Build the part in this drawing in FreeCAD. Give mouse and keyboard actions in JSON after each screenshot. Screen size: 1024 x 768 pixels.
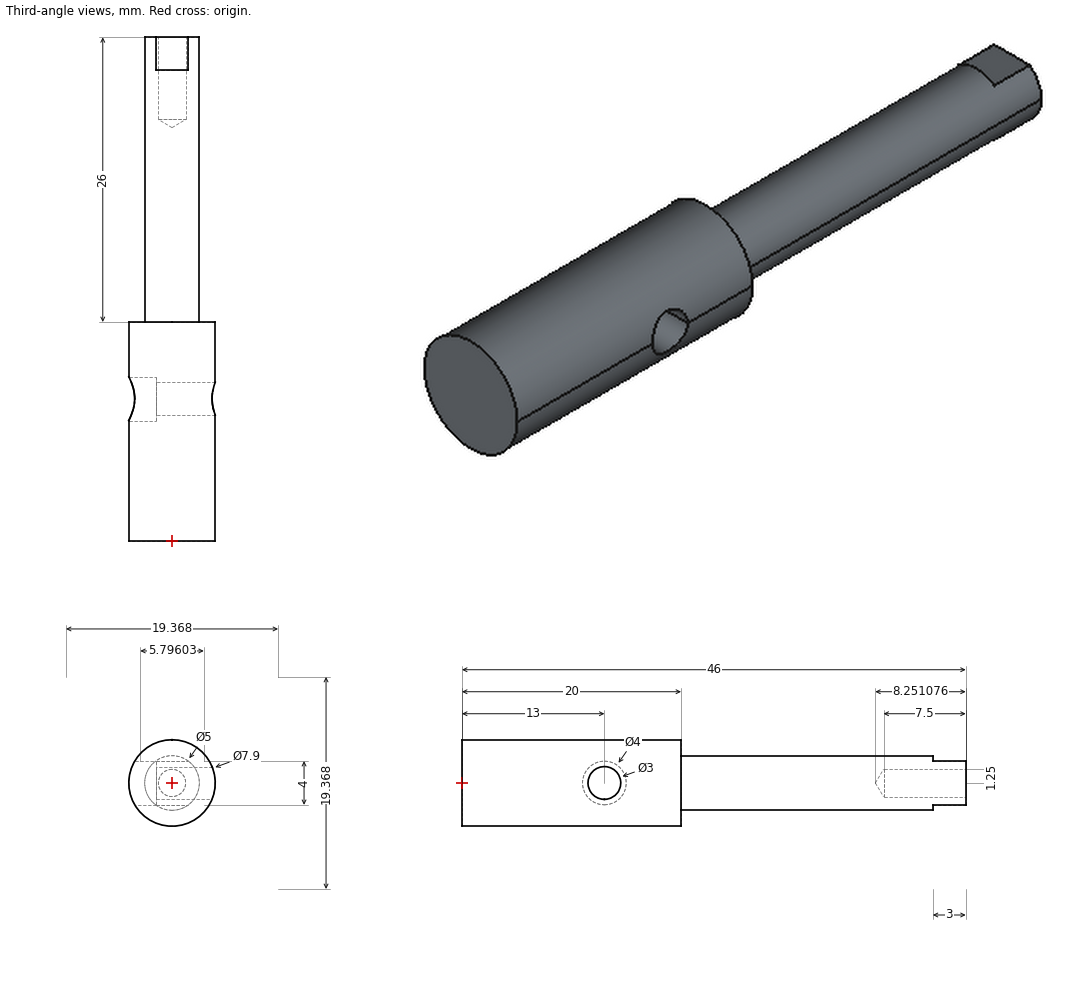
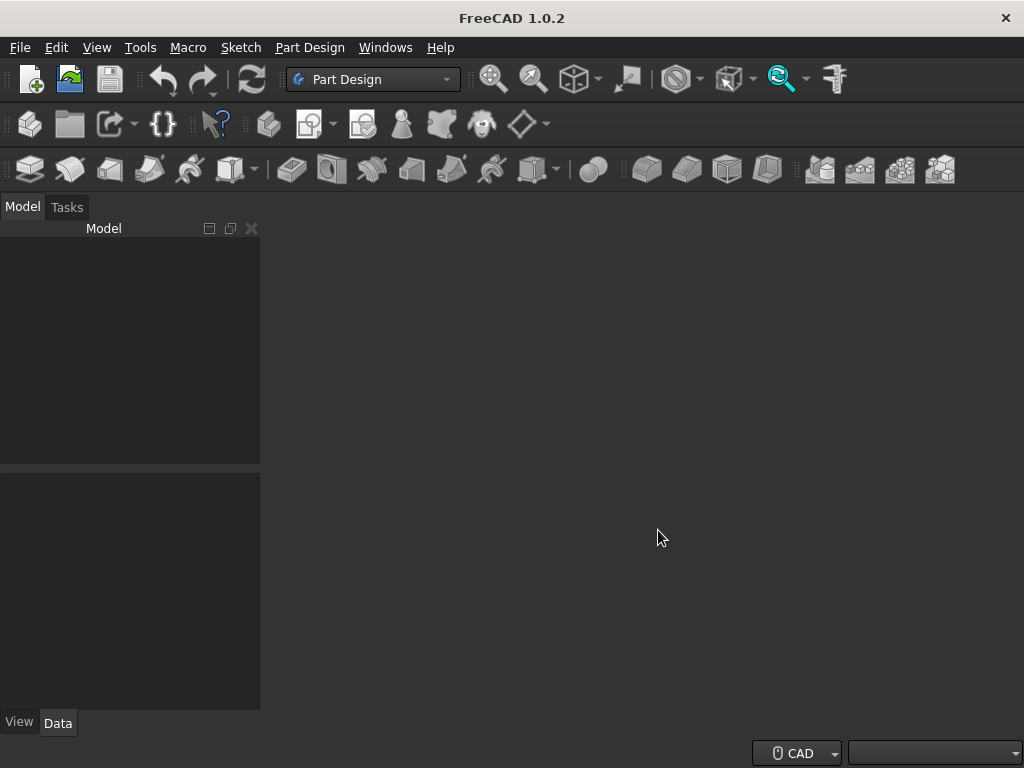
{"action": "left_click", "coordinate": [30, 80]}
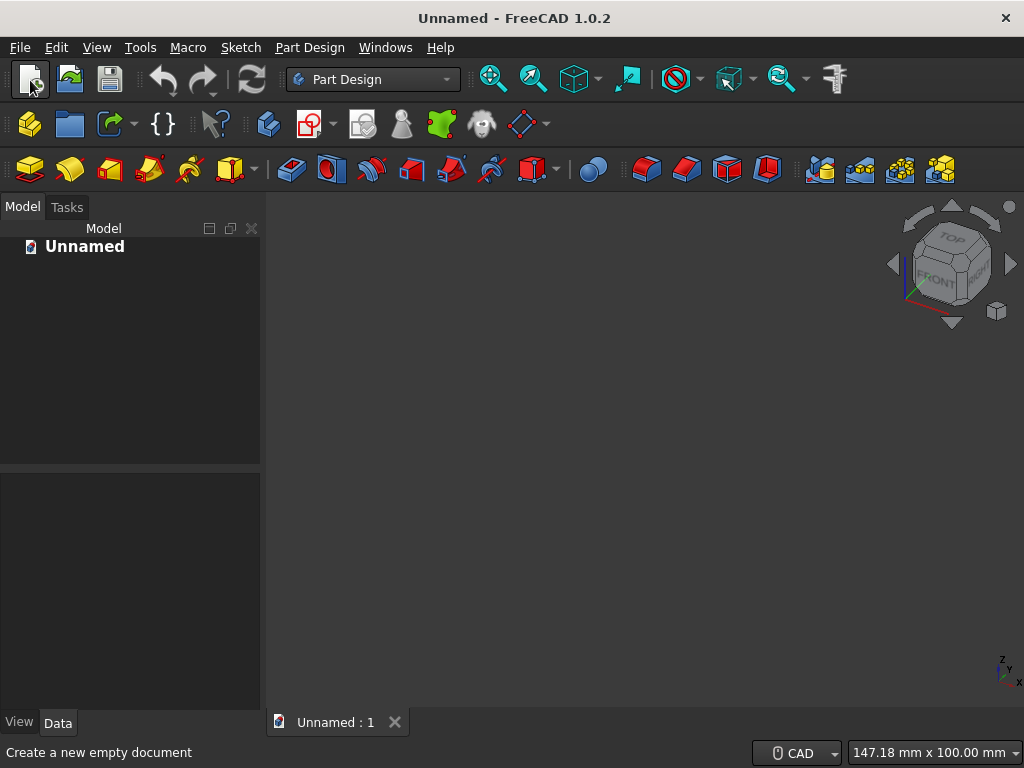
{"action": "left_click", "coordinate": [310, 124]}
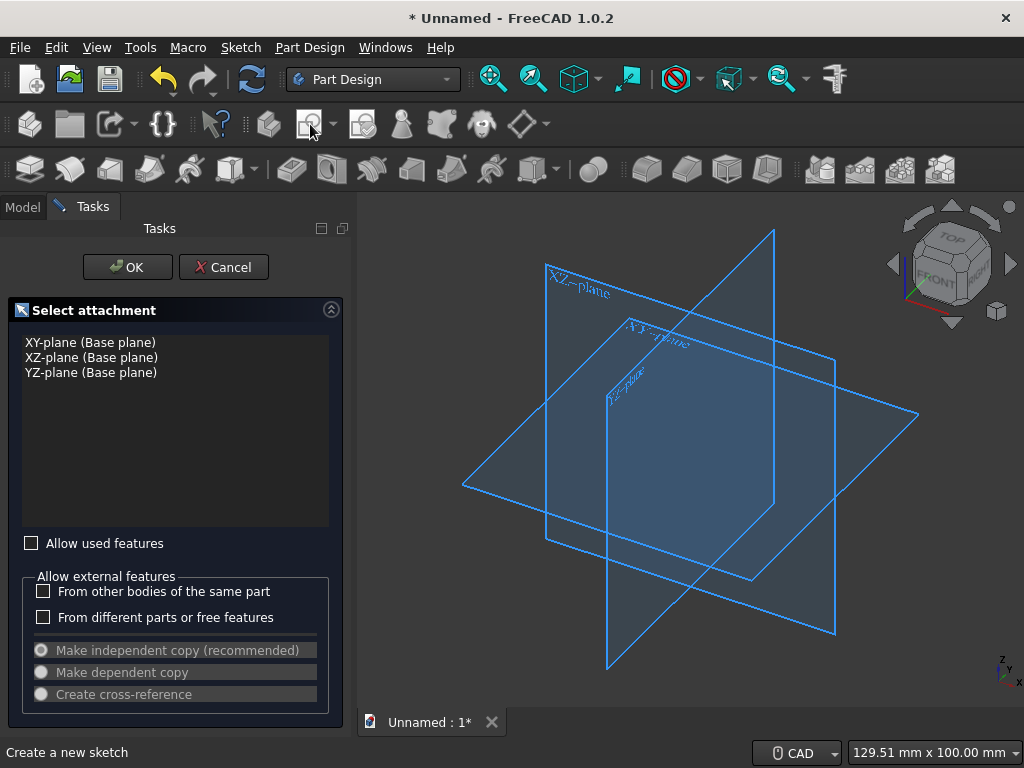
{"action": "left_click", "coordinate": [82, 358]}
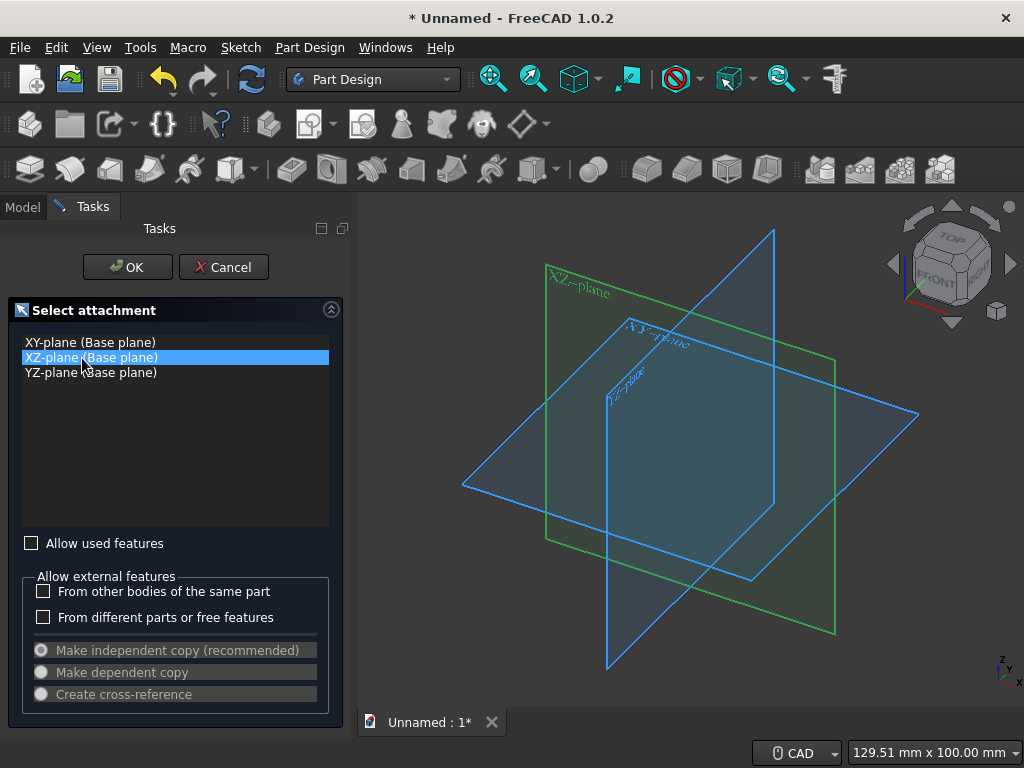
{"action": "left_click", "coordinate": [128, 267]}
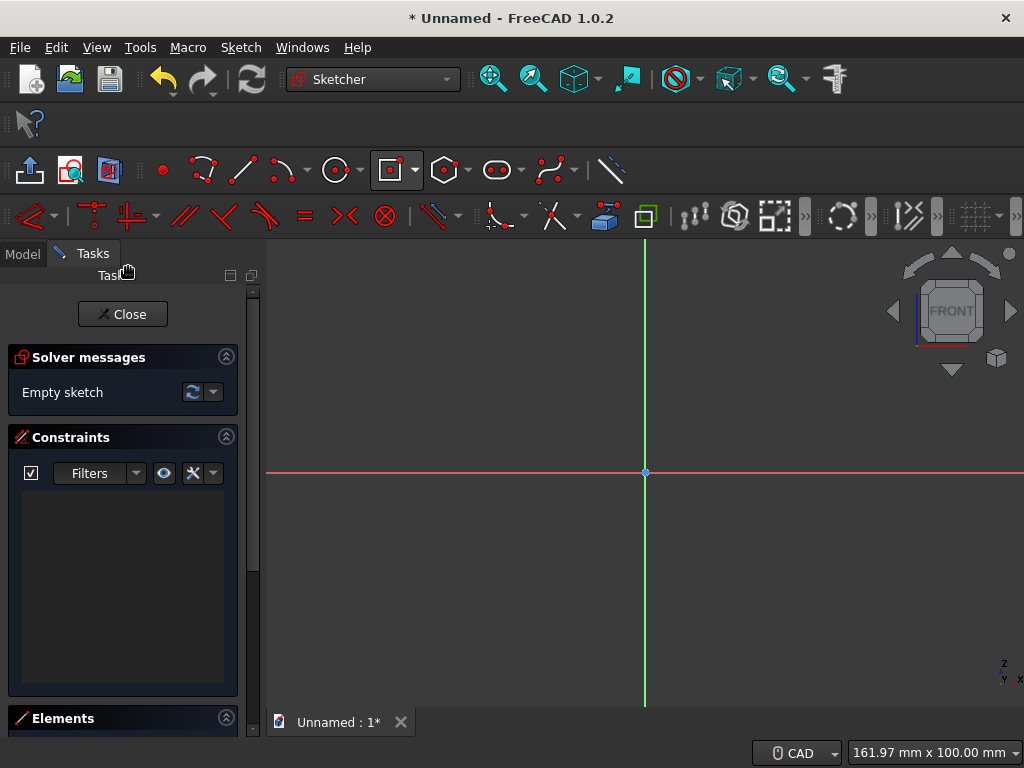
{"action": "scroll", "coordinate": [656, 473], "scroll_direction": "up", "scroll_amount": 10}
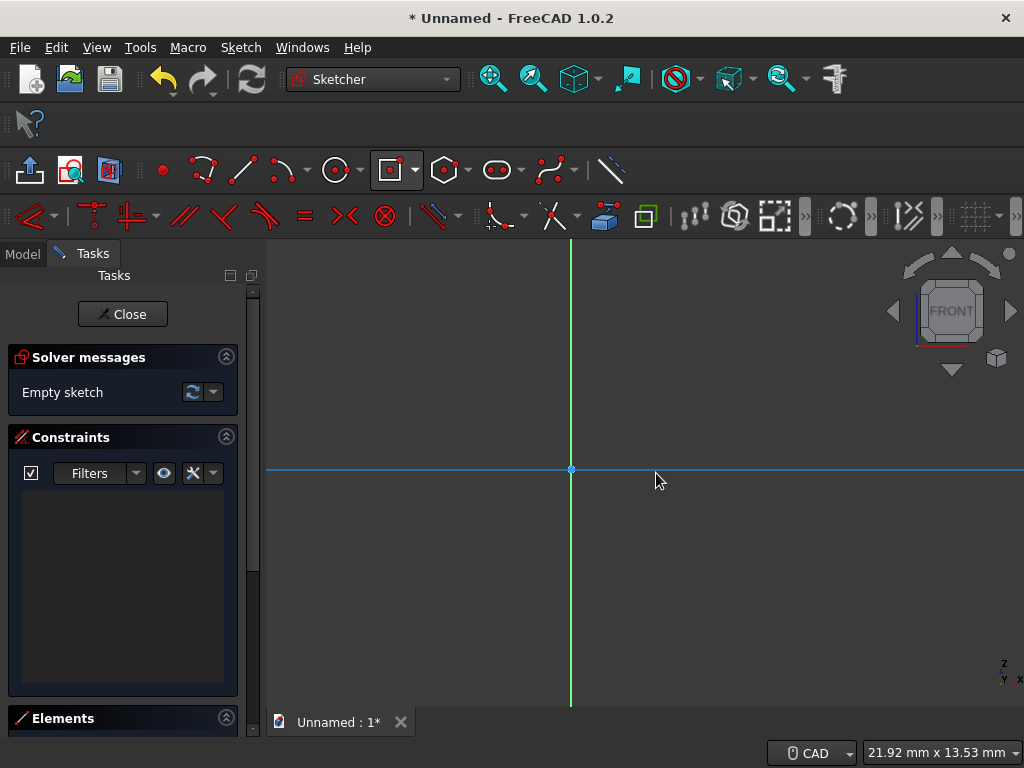
{"action": "left_click", "coordinate": [336, 170]}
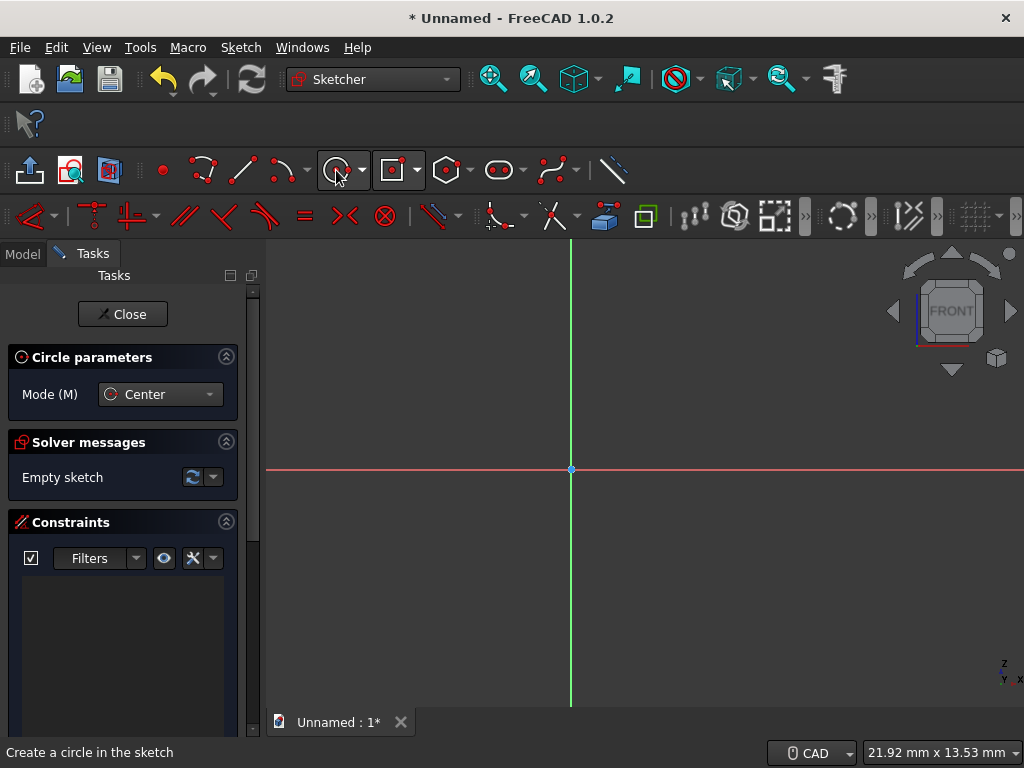
{"action": "left_click", "coordinate": [571, 470]}
{"action": "mouse_move", "coordinate": [668, 373]}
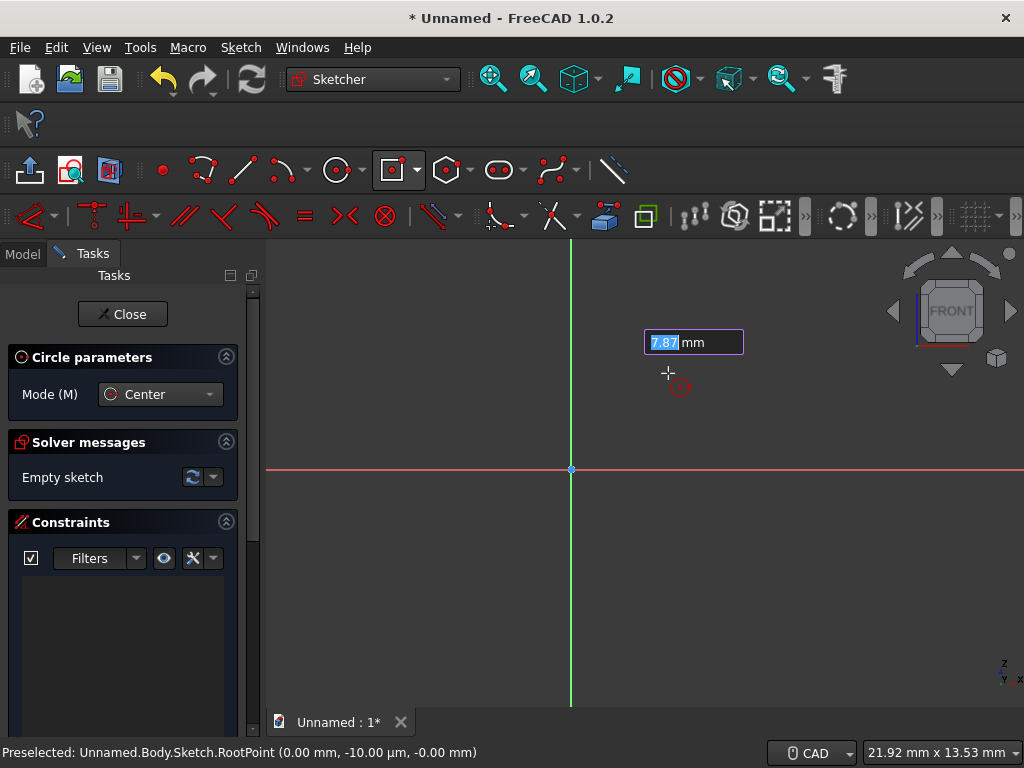
{"action": "type", "text": "7.9"}
{"action": "key", "text": "Return"}
{"action": "key", "text": "Escape"}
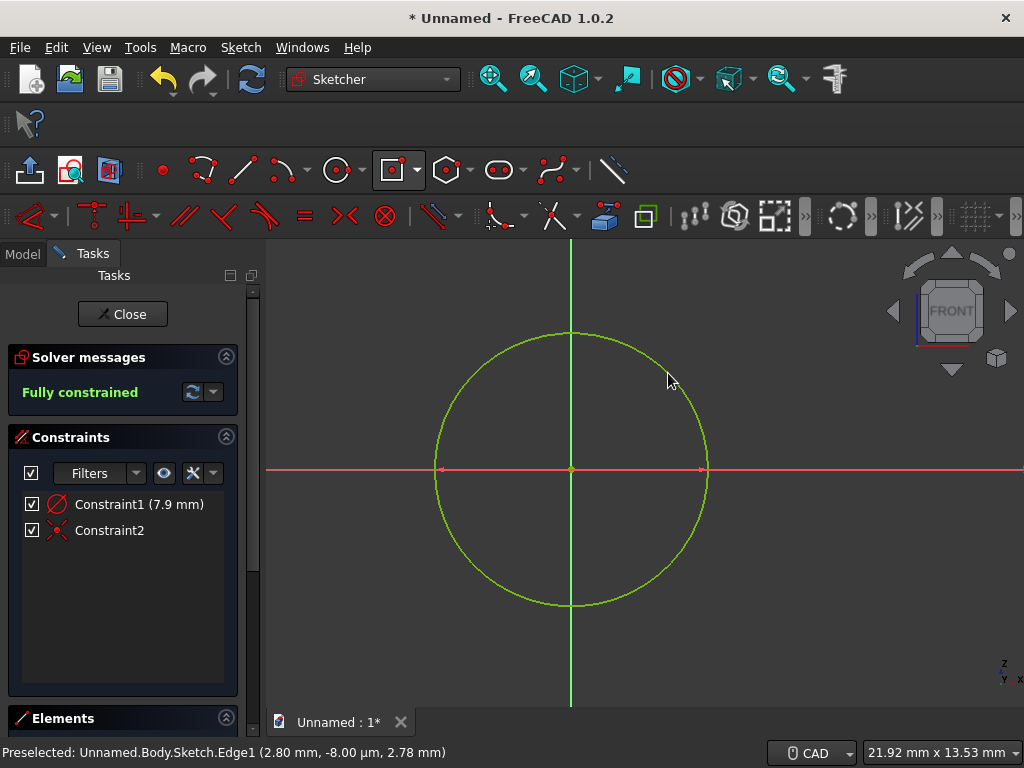
{"action": "left_click", "coordinate": [123, 314]}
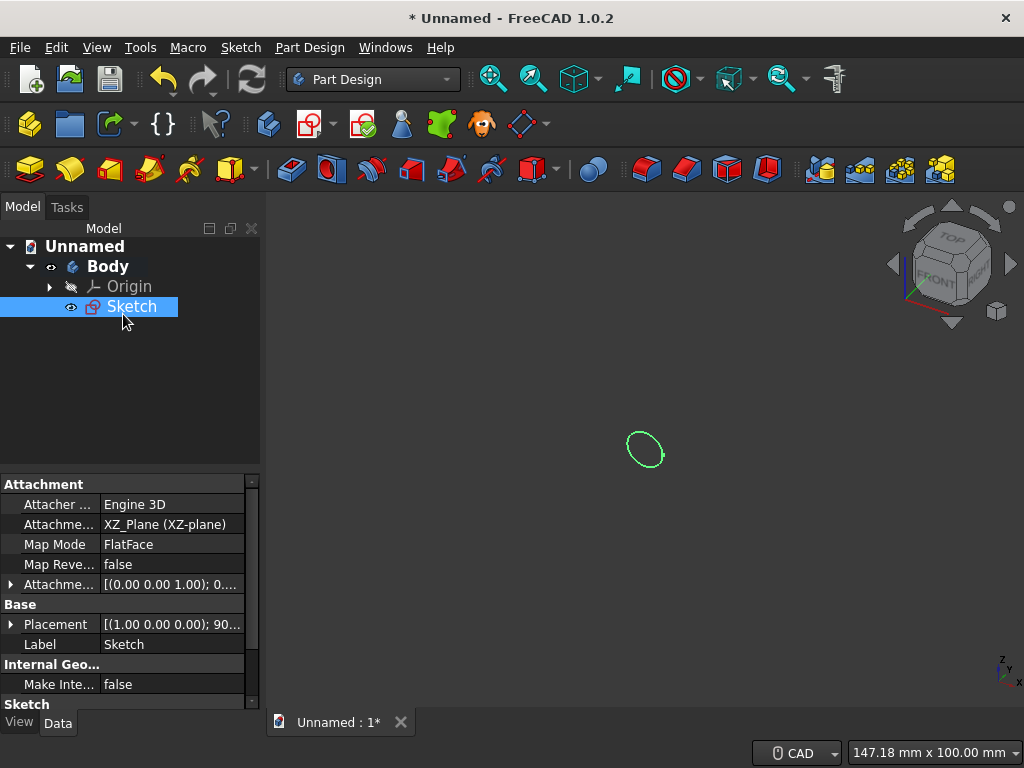
{"action": "left_click", "coordinate": [30, 170]}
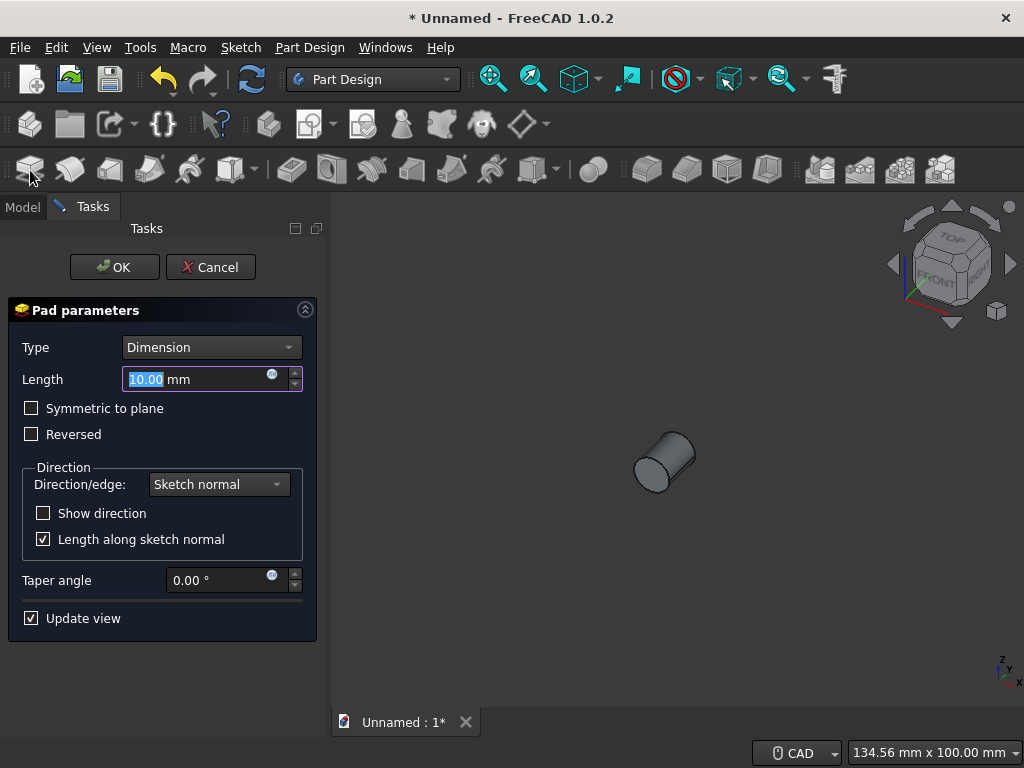
{"action": "type", "text": "20"}
{"action": "key", "text": "Tab"}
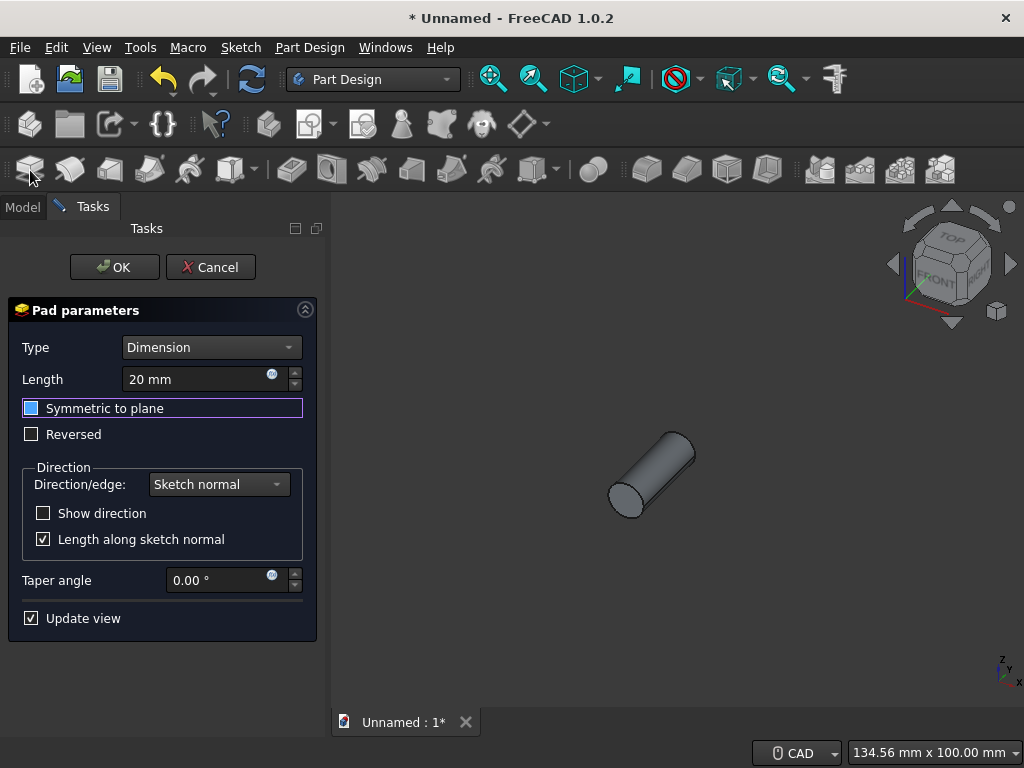
{"action": "left_click", "coordinate": [30, 434]}